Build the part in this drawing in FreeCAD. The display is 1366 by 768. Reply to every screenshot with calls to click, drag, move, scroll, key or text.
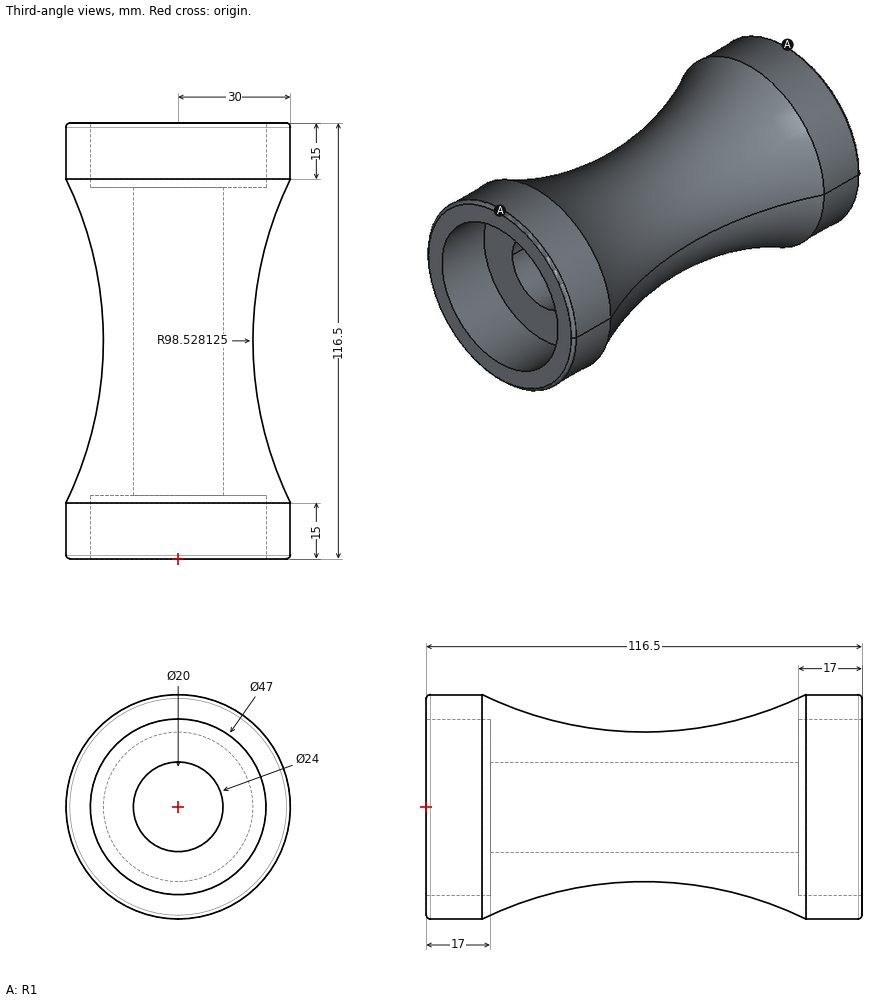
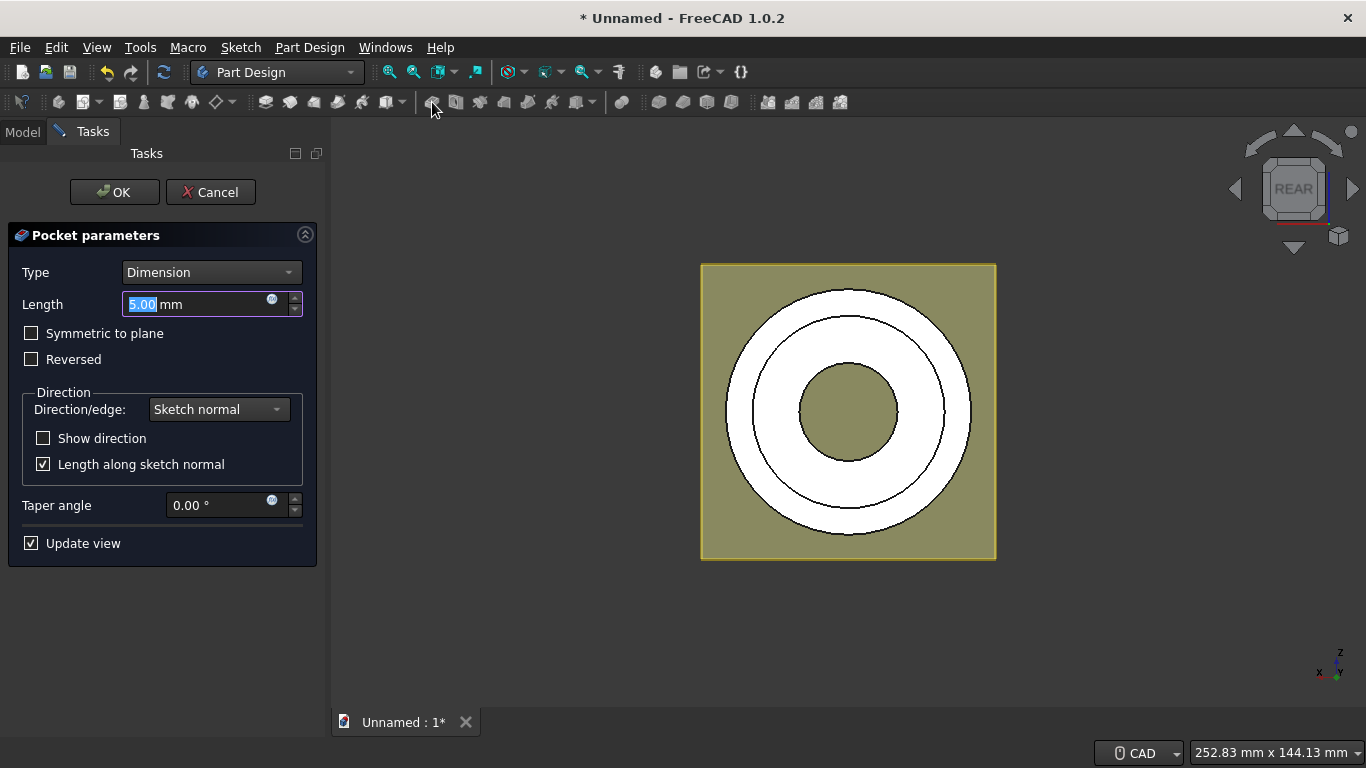
text(17)
key(Tab)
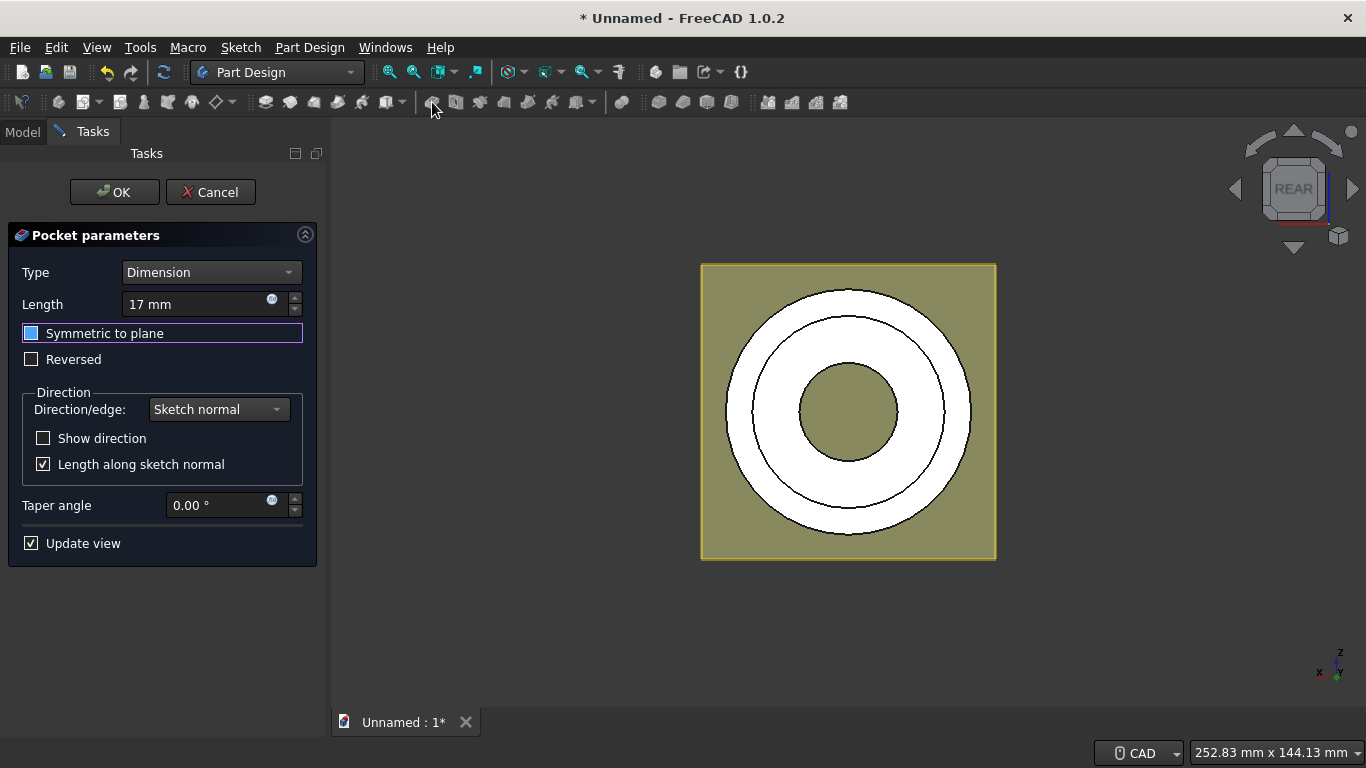
click(30, 359)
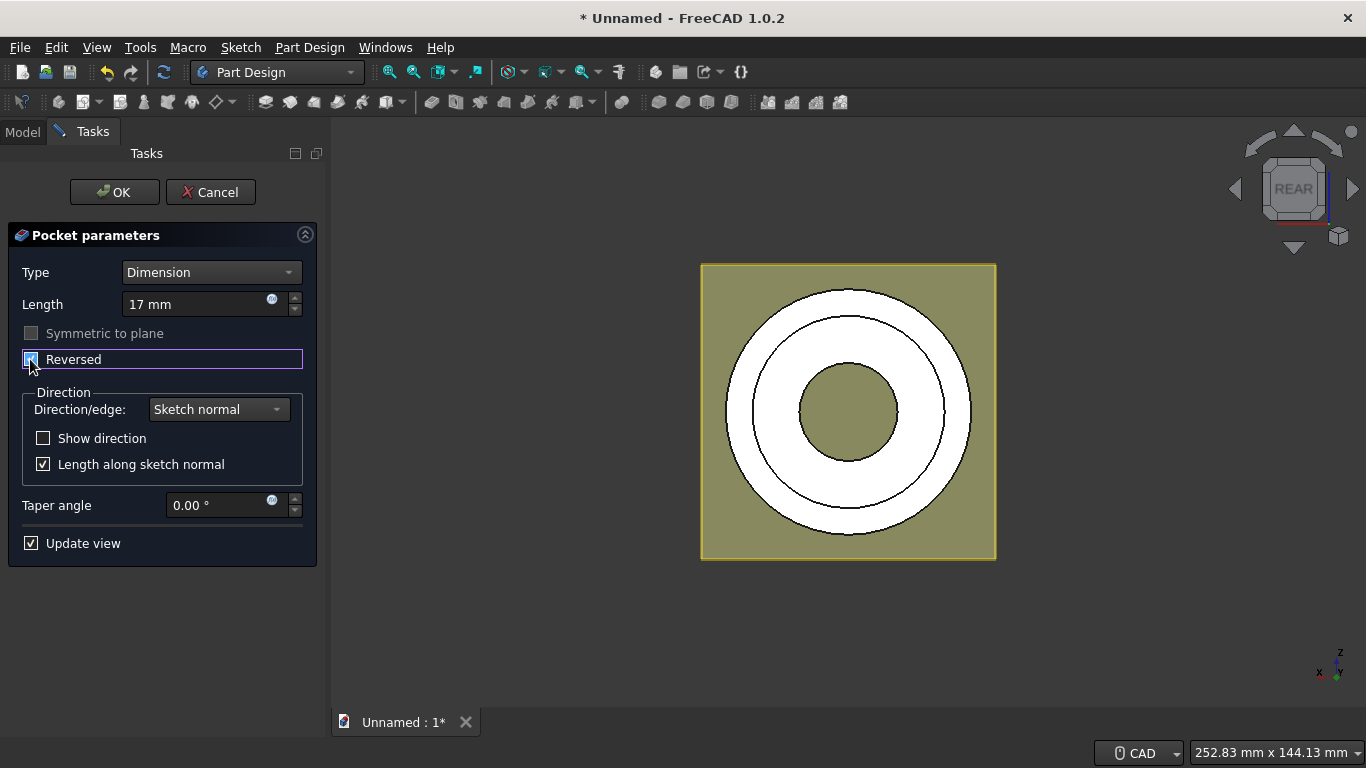
click(115, 192)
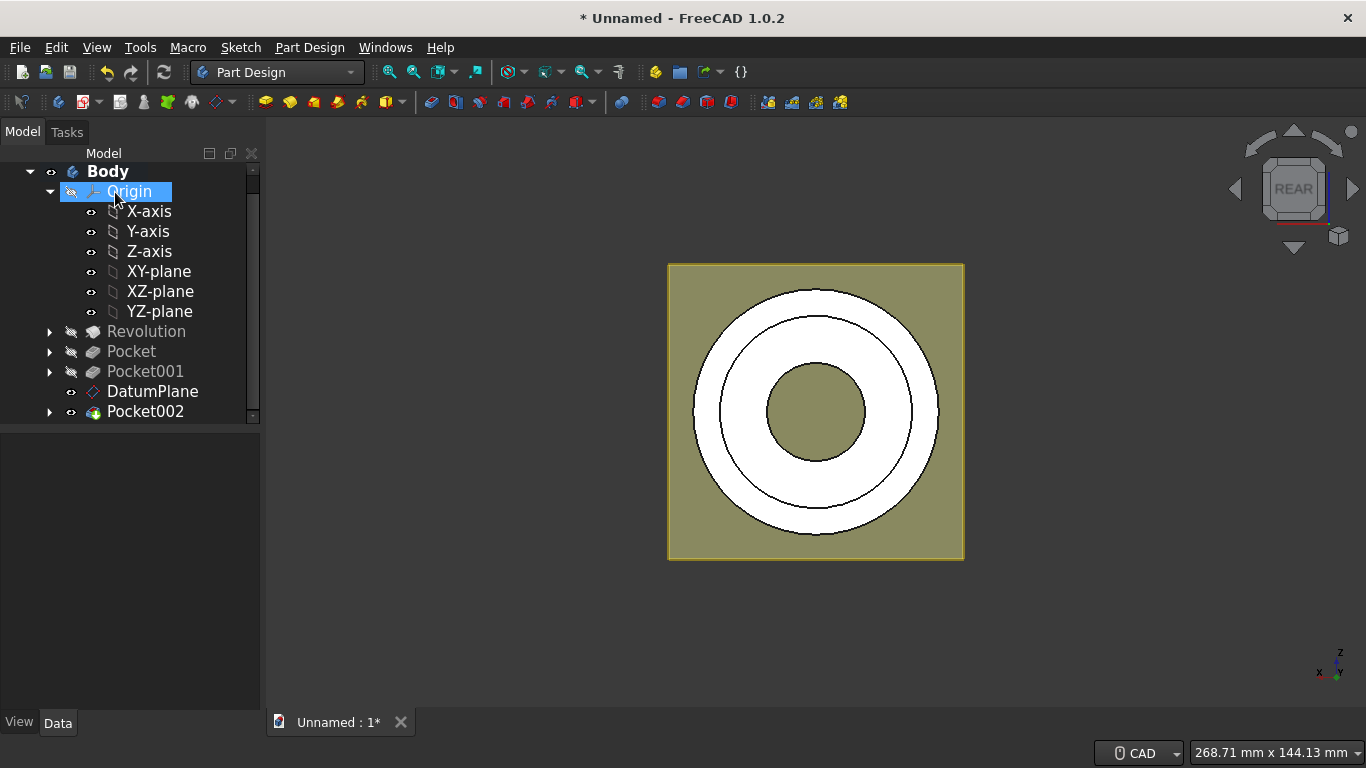
click(116, 392)
key(space)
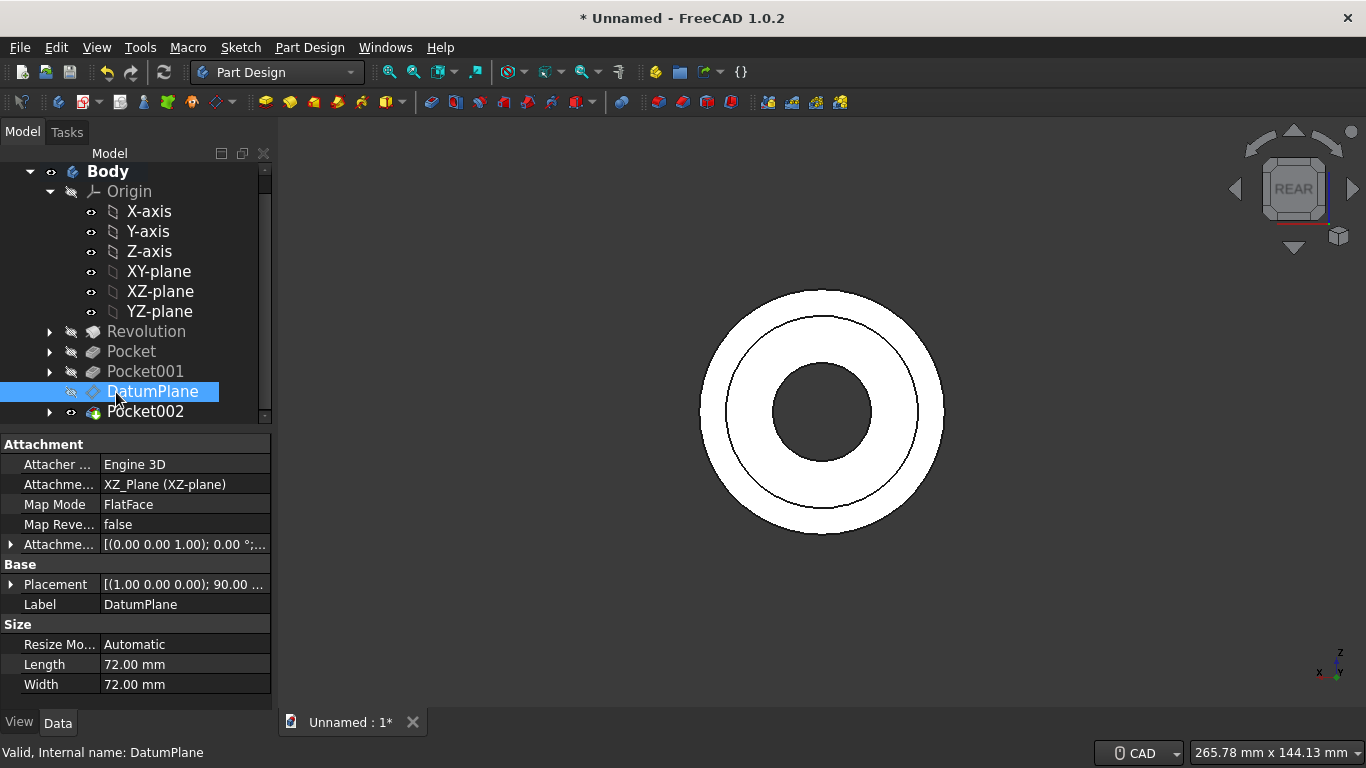
click(390, 72)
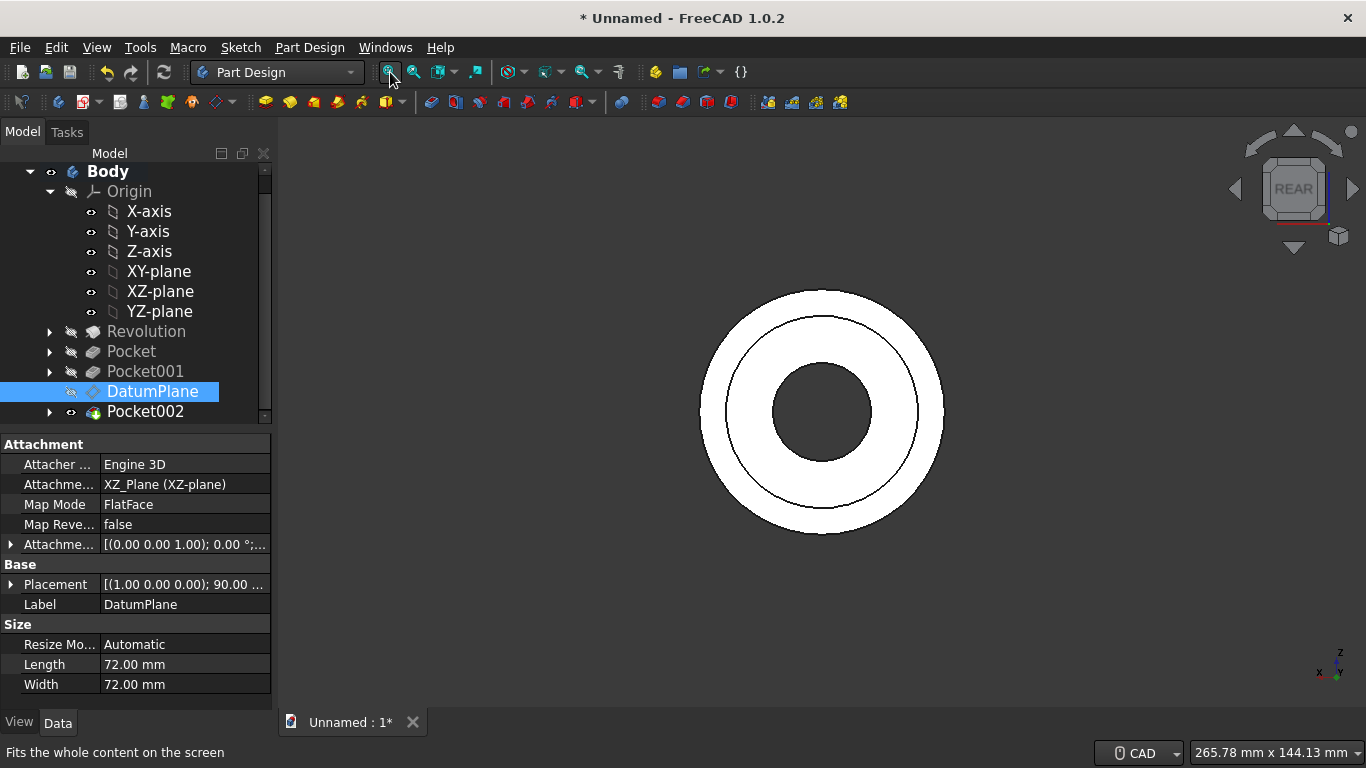
click(945, 411)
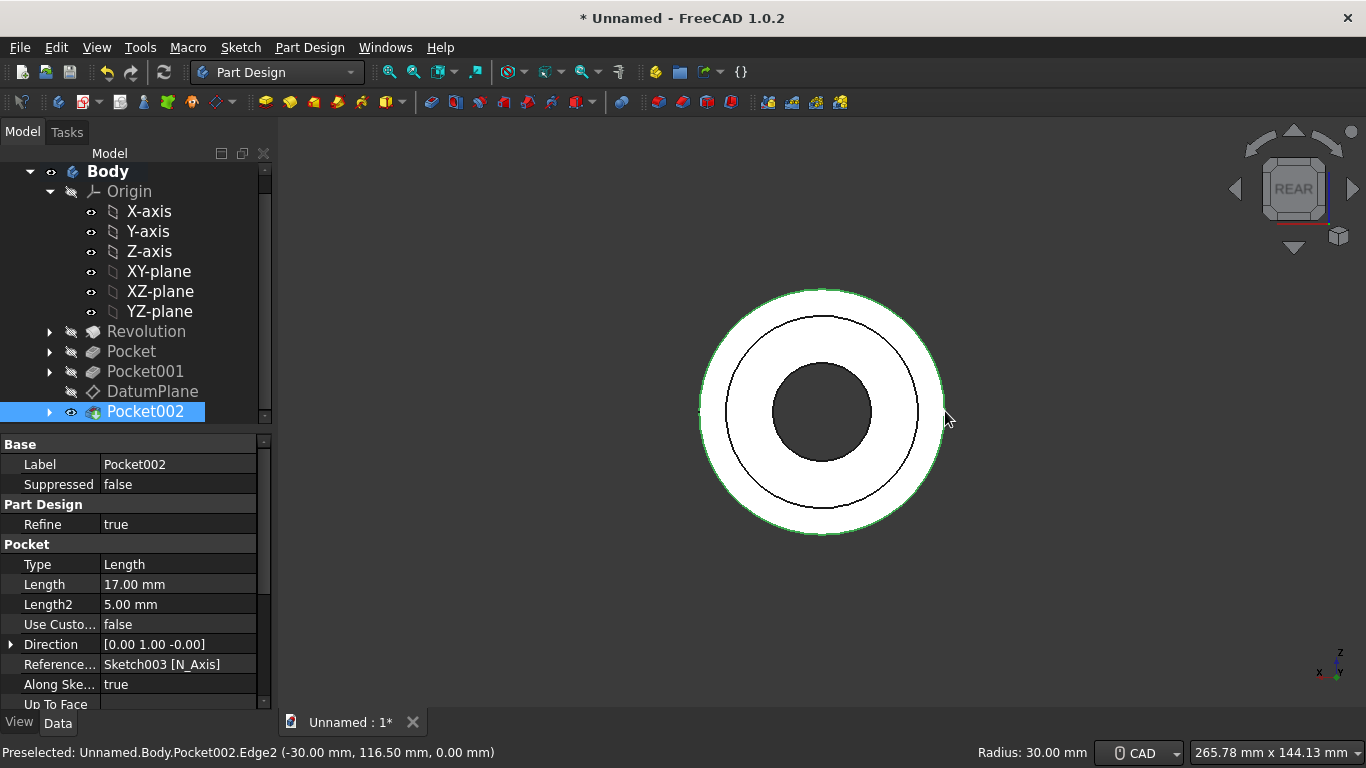
key(0)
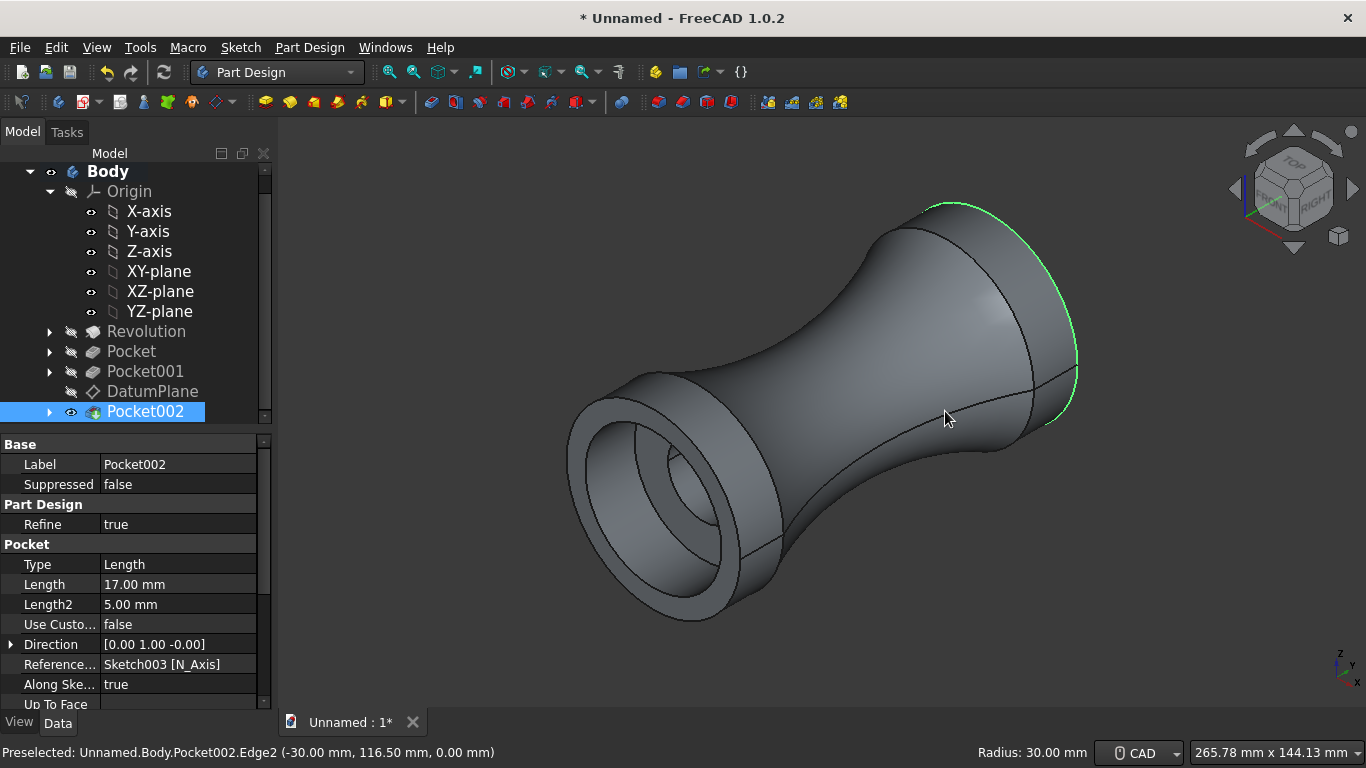
click(627, 397, ctrl)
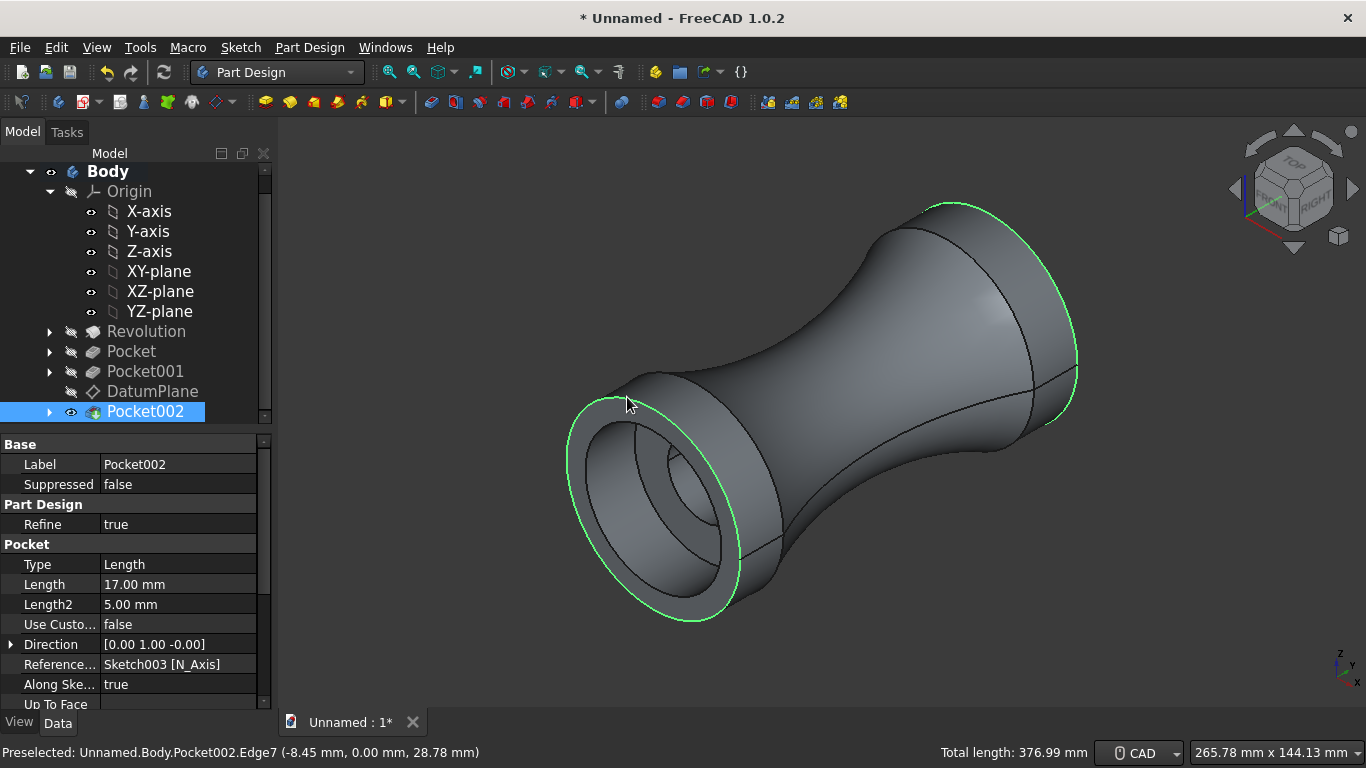
click(660, 102)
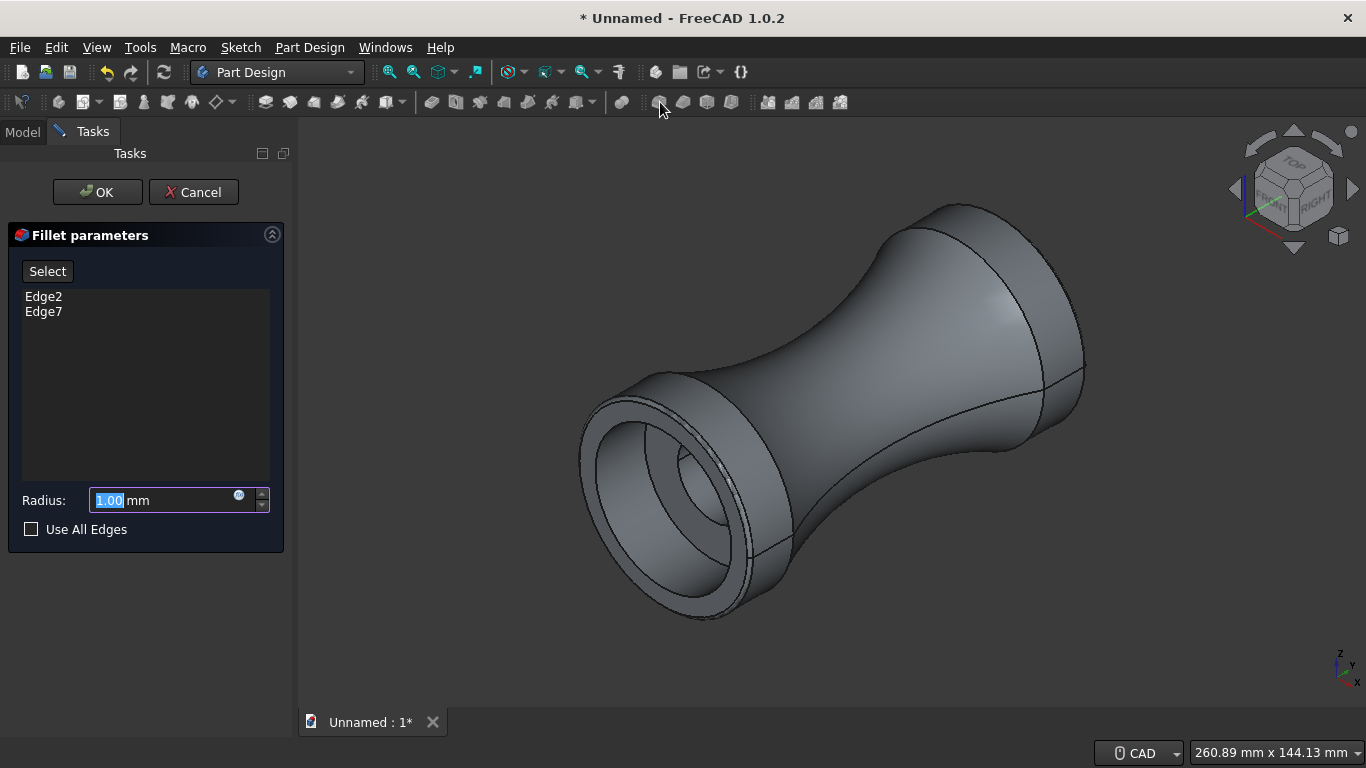
text(1)
key(Tab)